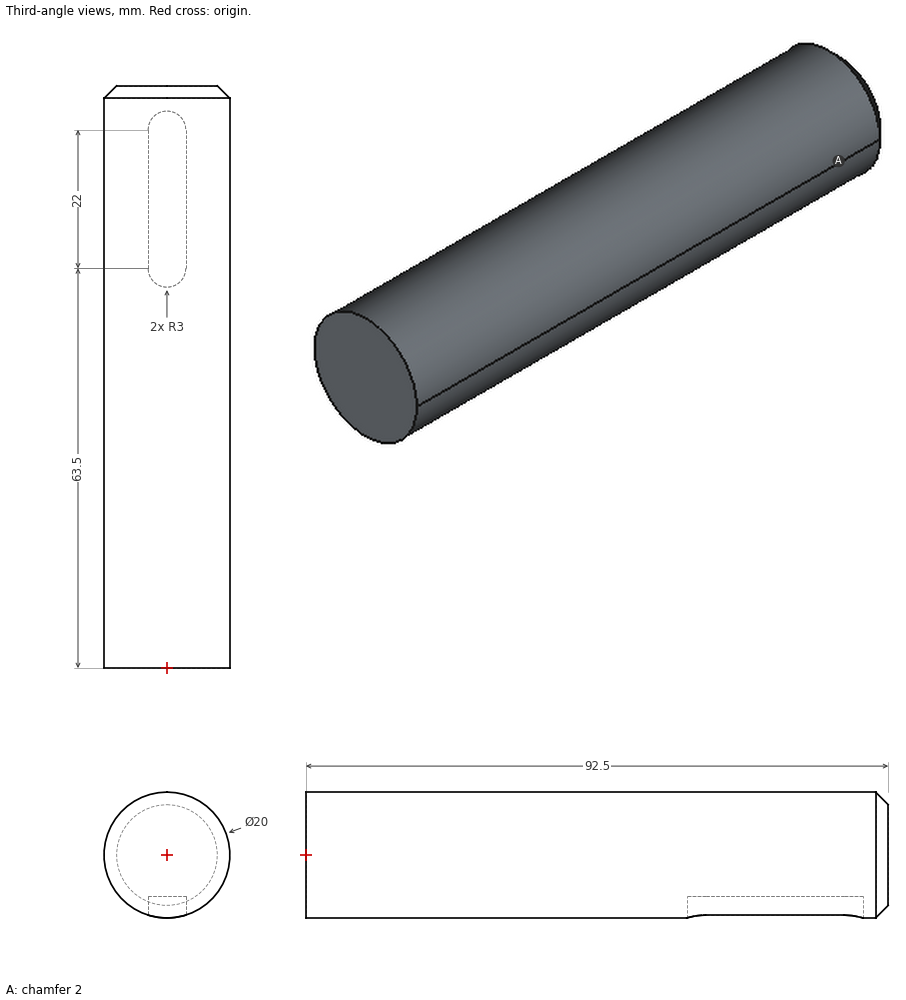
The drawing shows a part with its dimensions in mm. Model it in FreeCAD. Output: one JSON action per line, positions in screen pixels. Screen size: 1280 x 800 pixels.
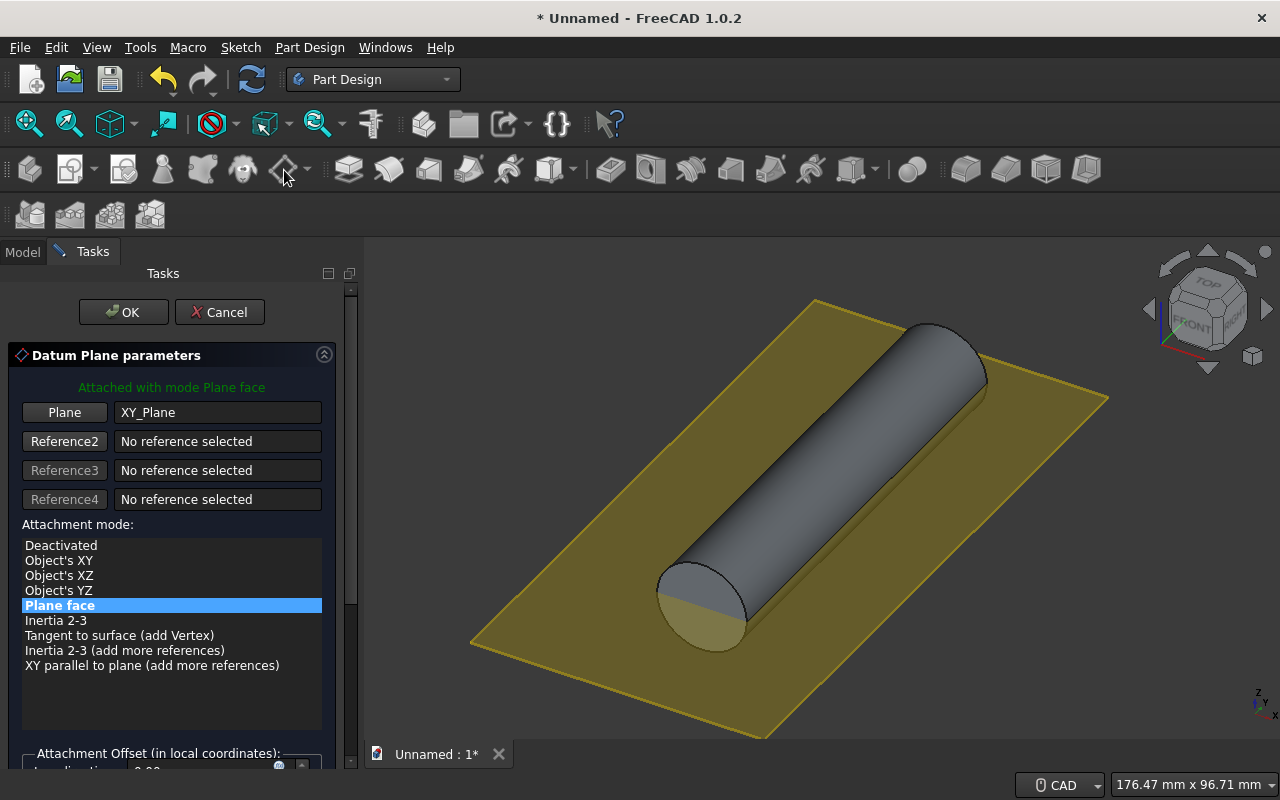
{"action": "scroll", "coordinate": [351, 526], "scroll_direction": "down", "scroll_amount": 3}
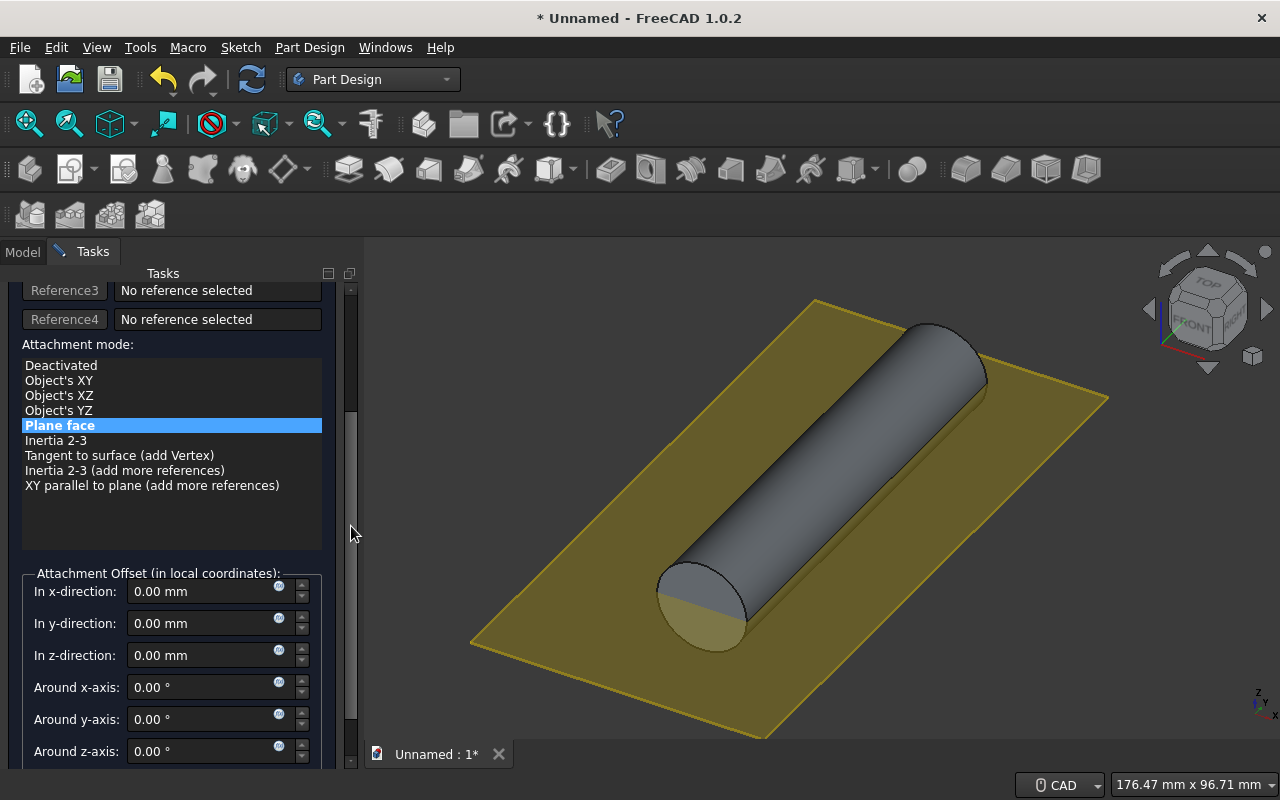
{"action": "triple_click", "coordinate": [210, 655]}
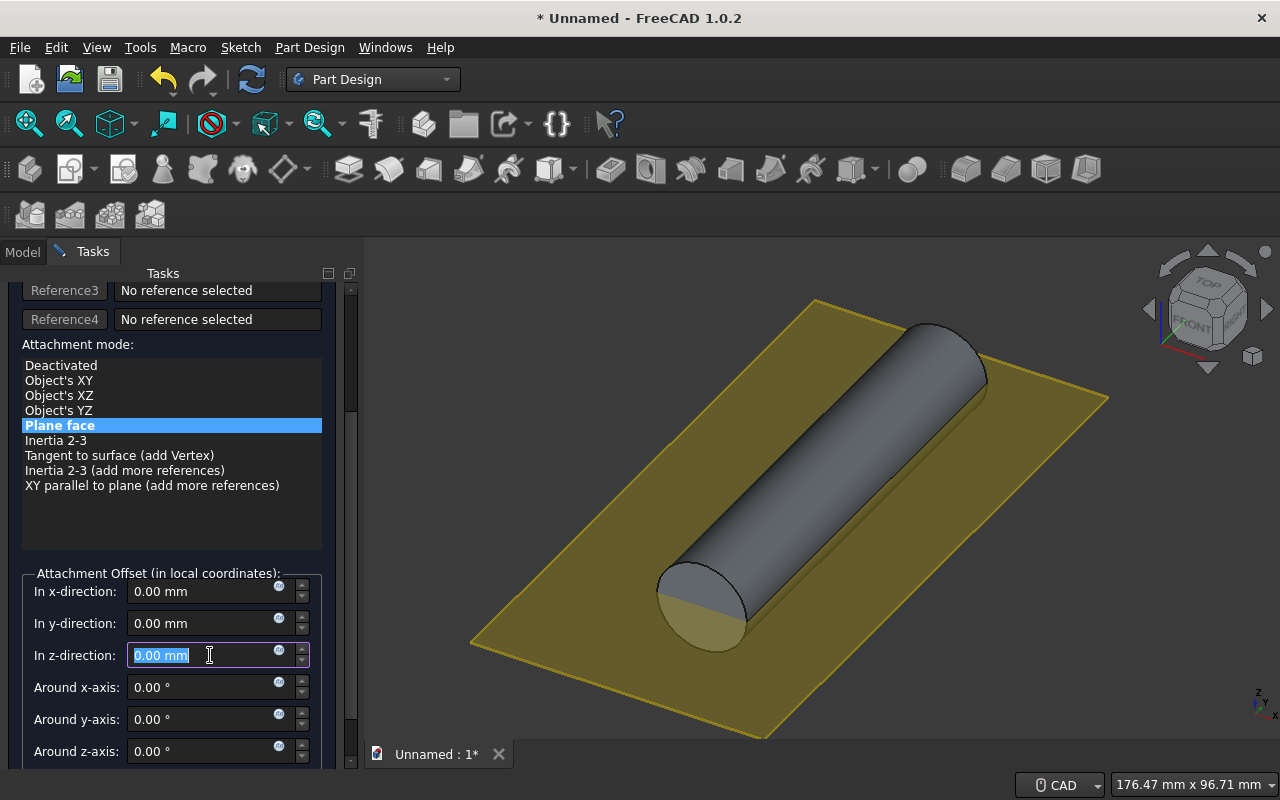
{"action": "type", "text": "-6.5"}
{"action": "key", "text": "Tab"}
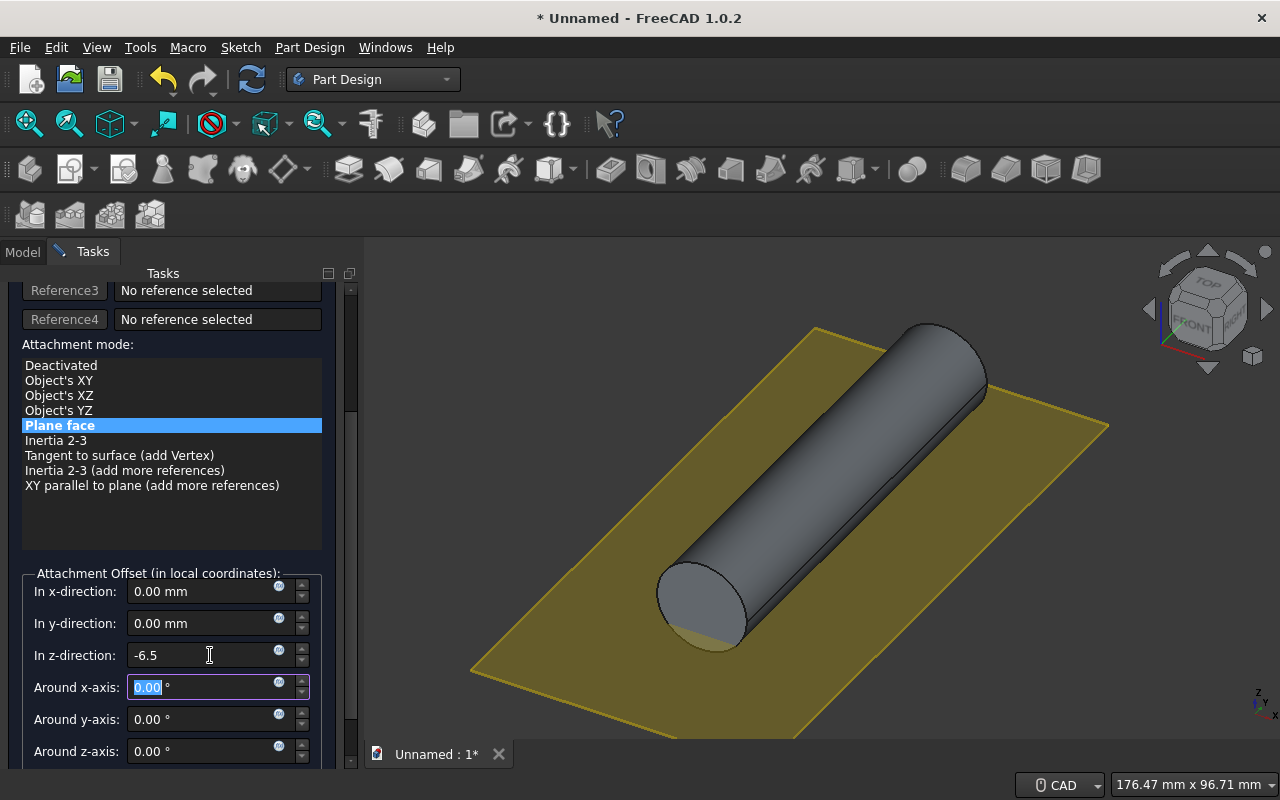
{"action": "scroll", "coordinate": [351, 526], "scroll_direction": "up", "scroll_amount": 4}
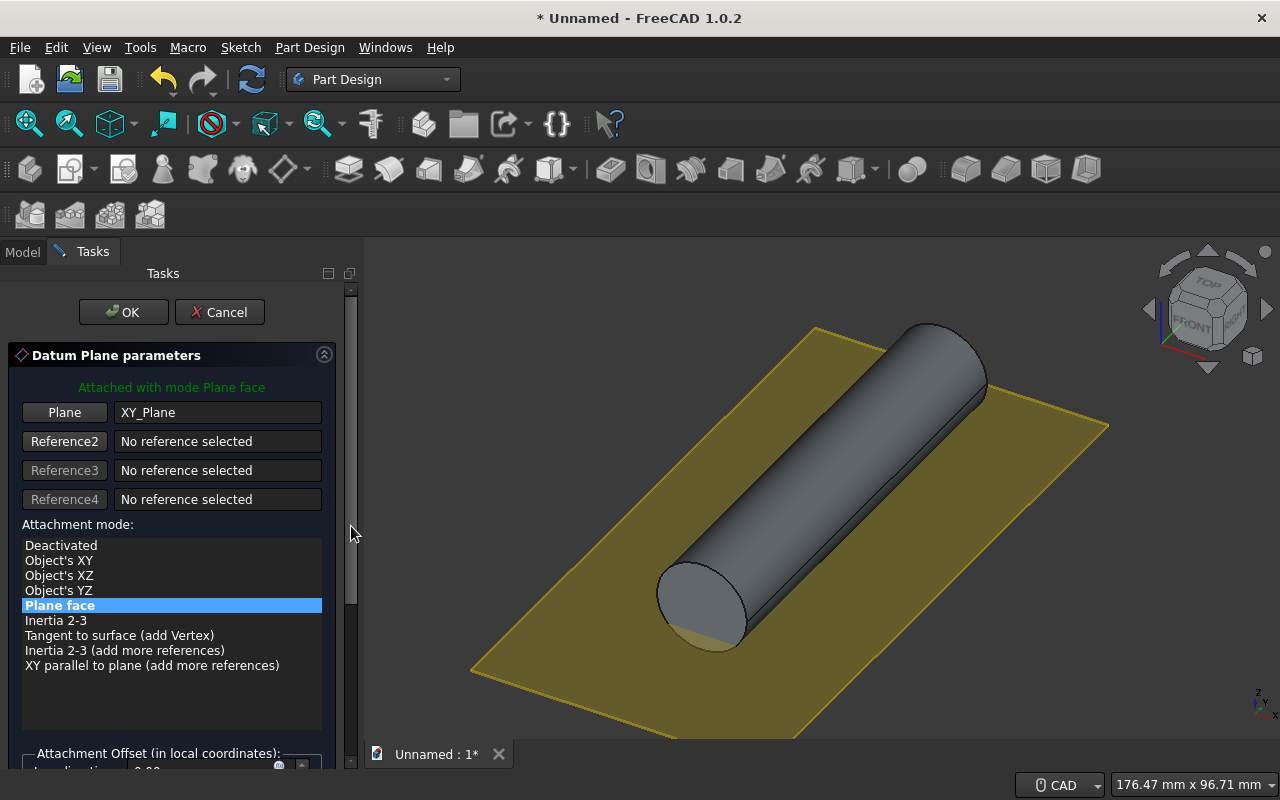
{"action": "left_click", "coordinate": [124, 312]}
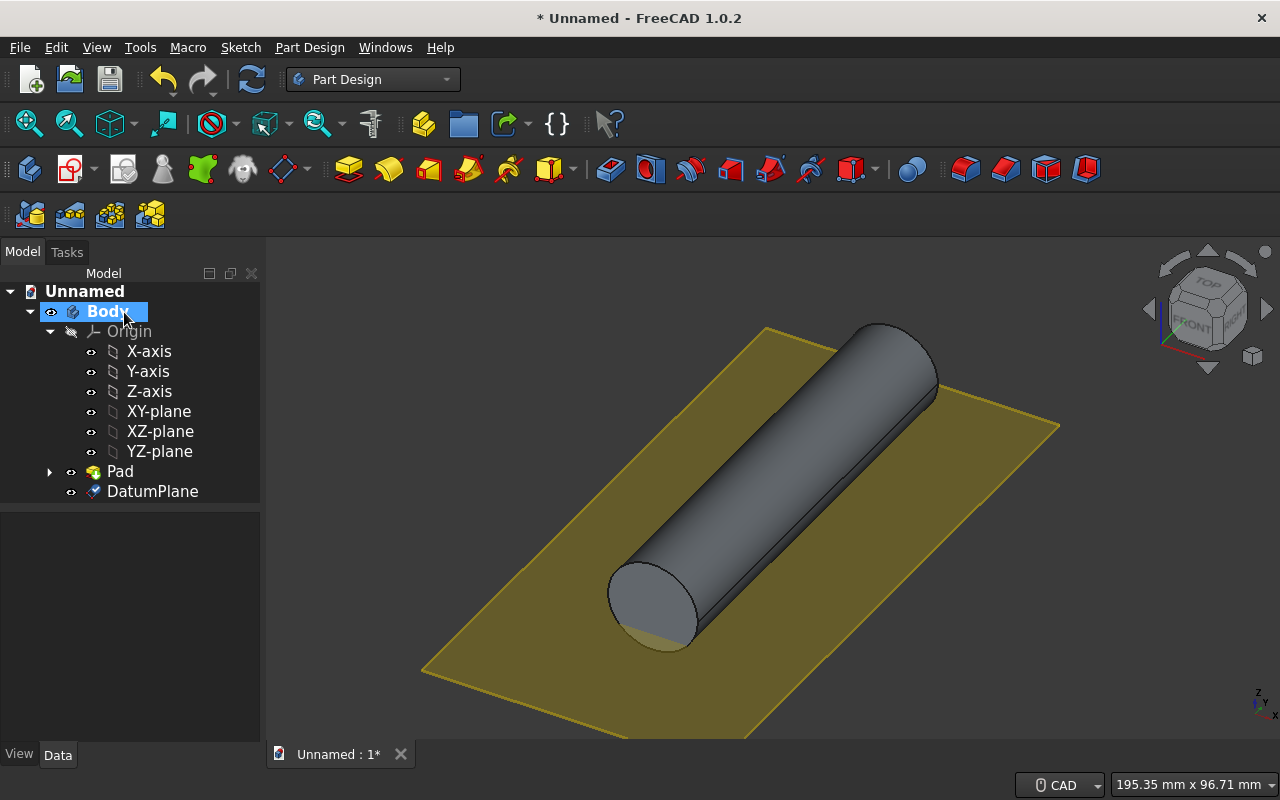
{"action": "left_click", "coordinate": [116, 492]}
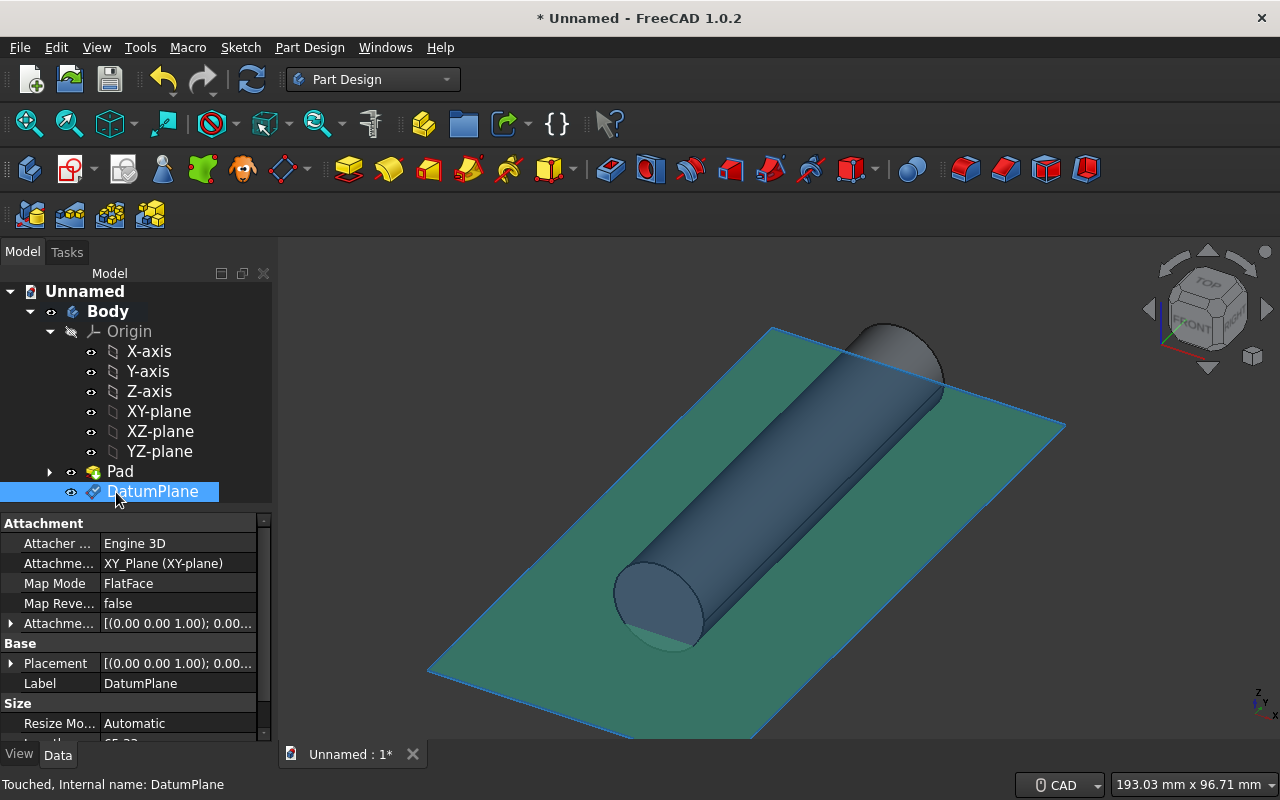
{"action": "left_click", "coordinate": [70, 170]}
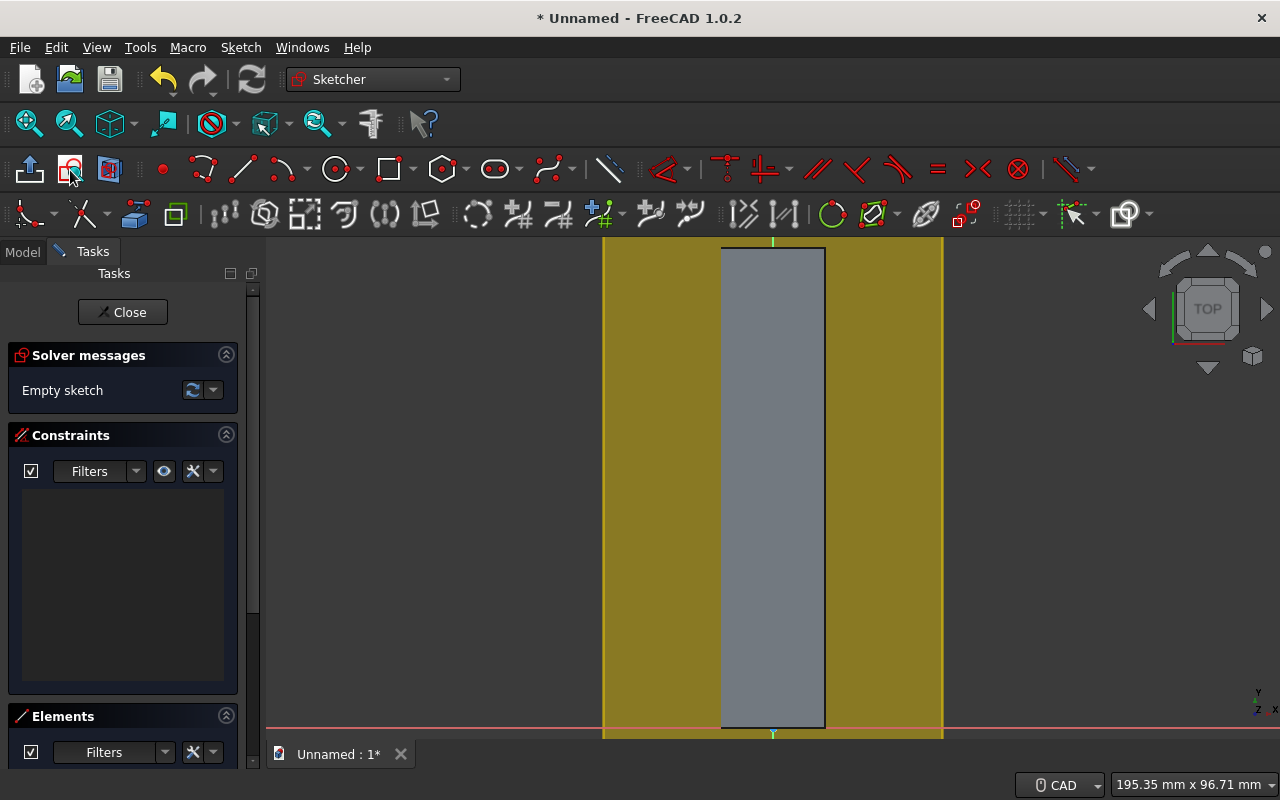
{"action": "key", "text": "q s"}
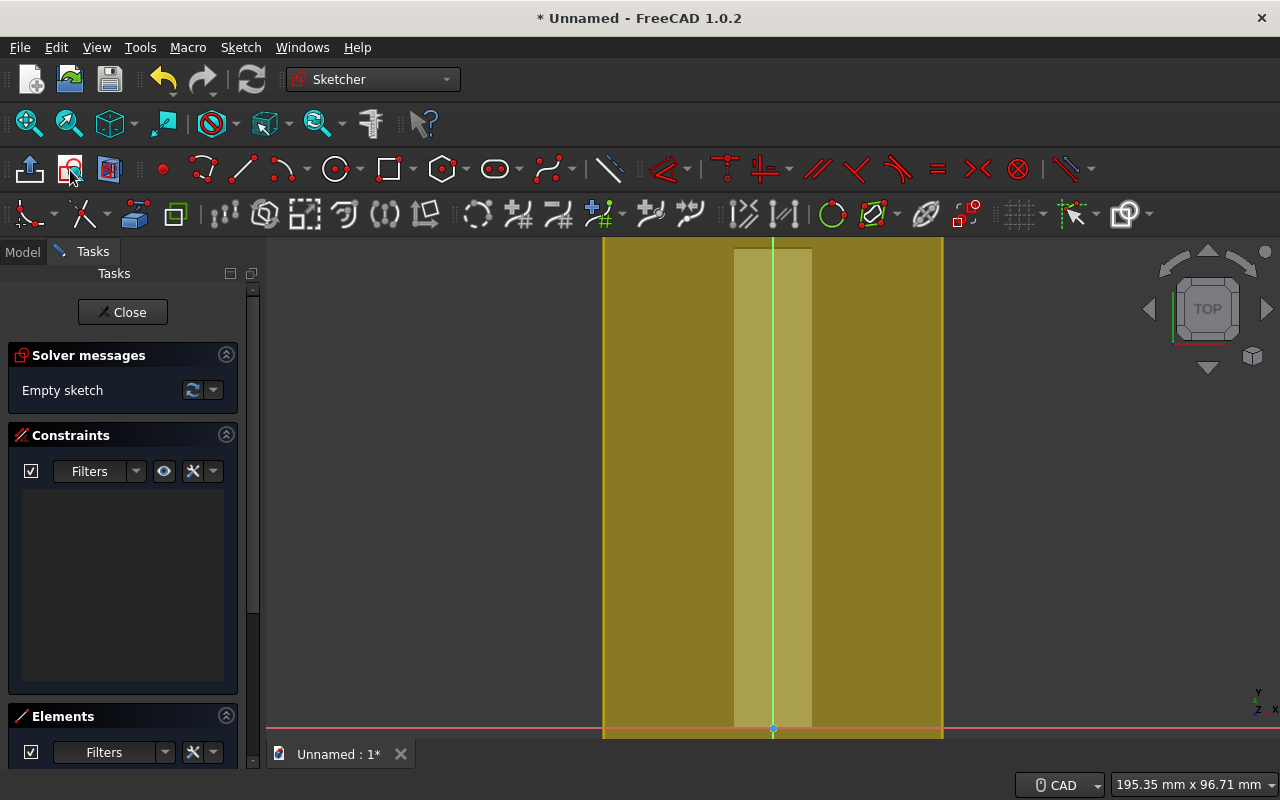
{"action": "scroll", "coordinate": [704, 488], "scroll_direction": "down", "scroll_amount": 5}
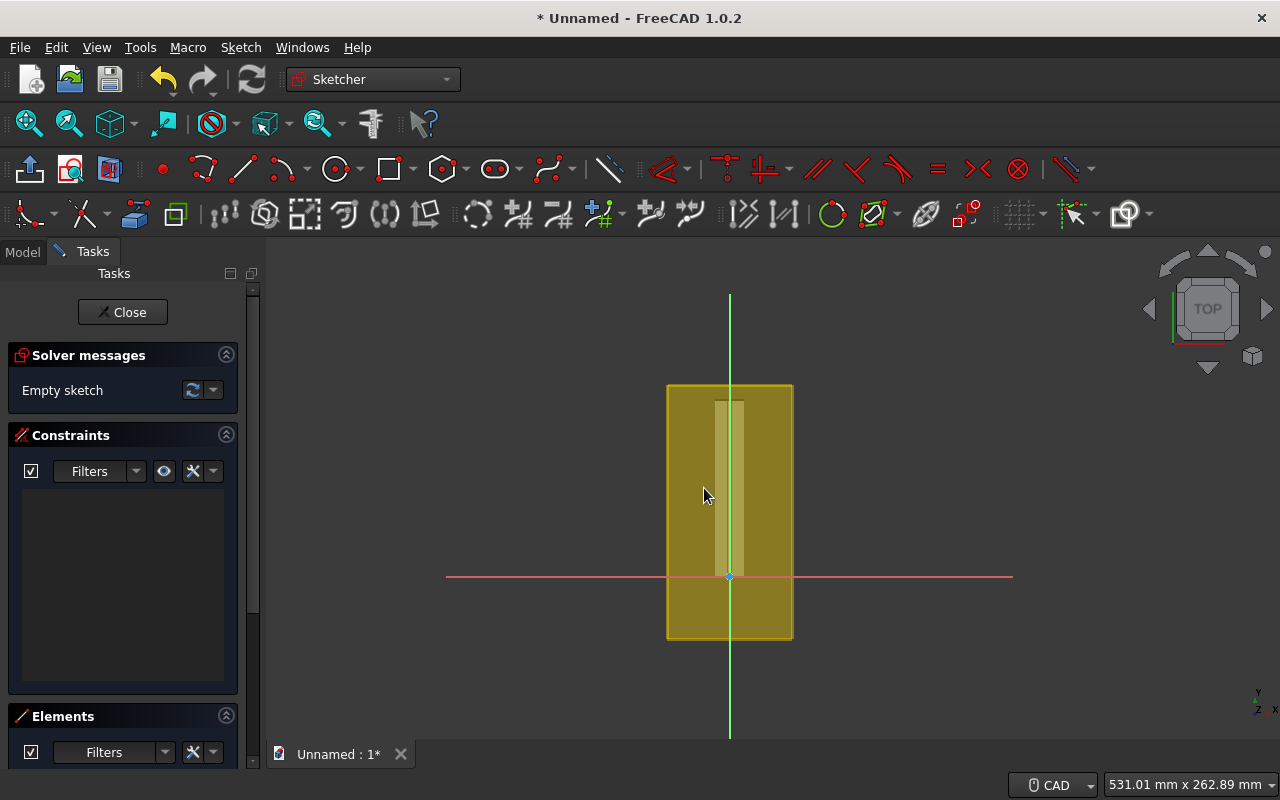
{"action": "scroll", "coordinate": [735, 424], "scroll_direction": "up", "scroll_amount": 9}